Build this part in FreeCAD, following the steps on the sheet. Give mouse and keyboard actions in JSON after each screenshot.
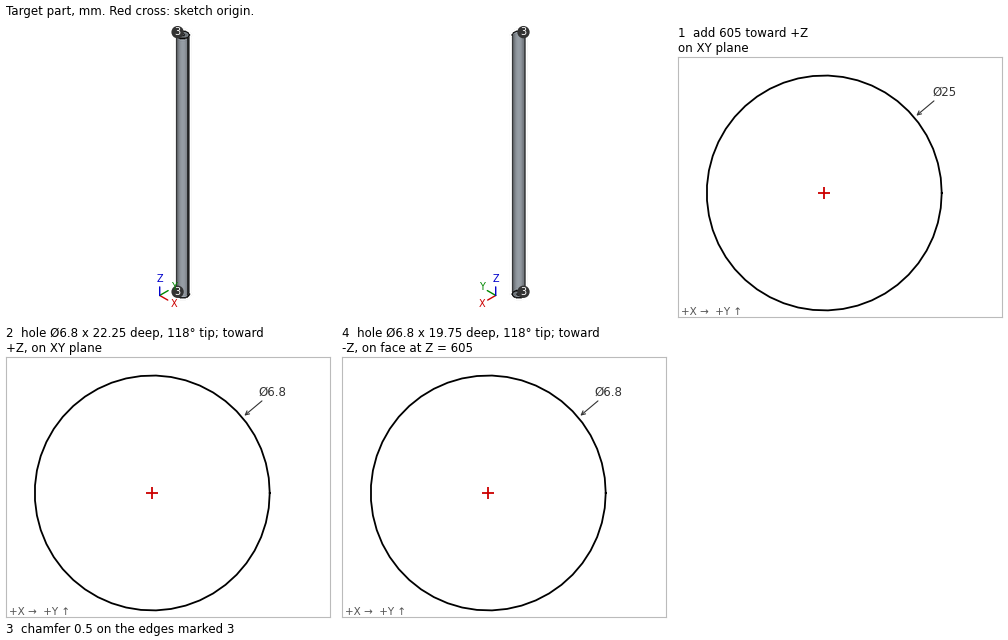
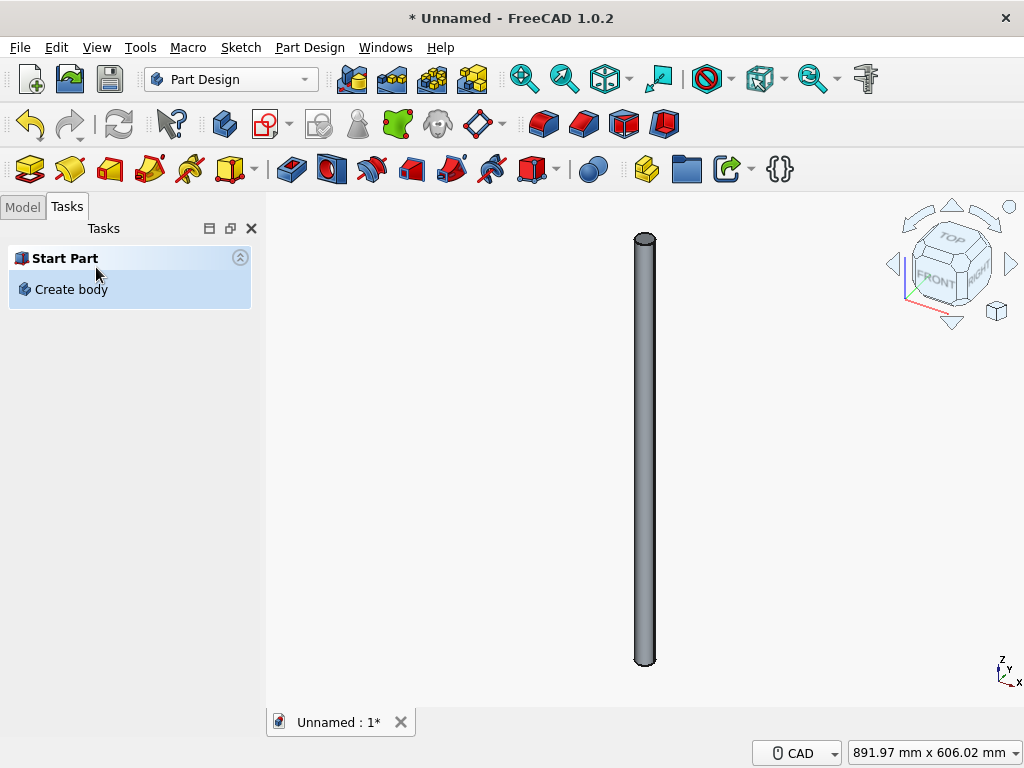
{"action": "key", "text": "0"}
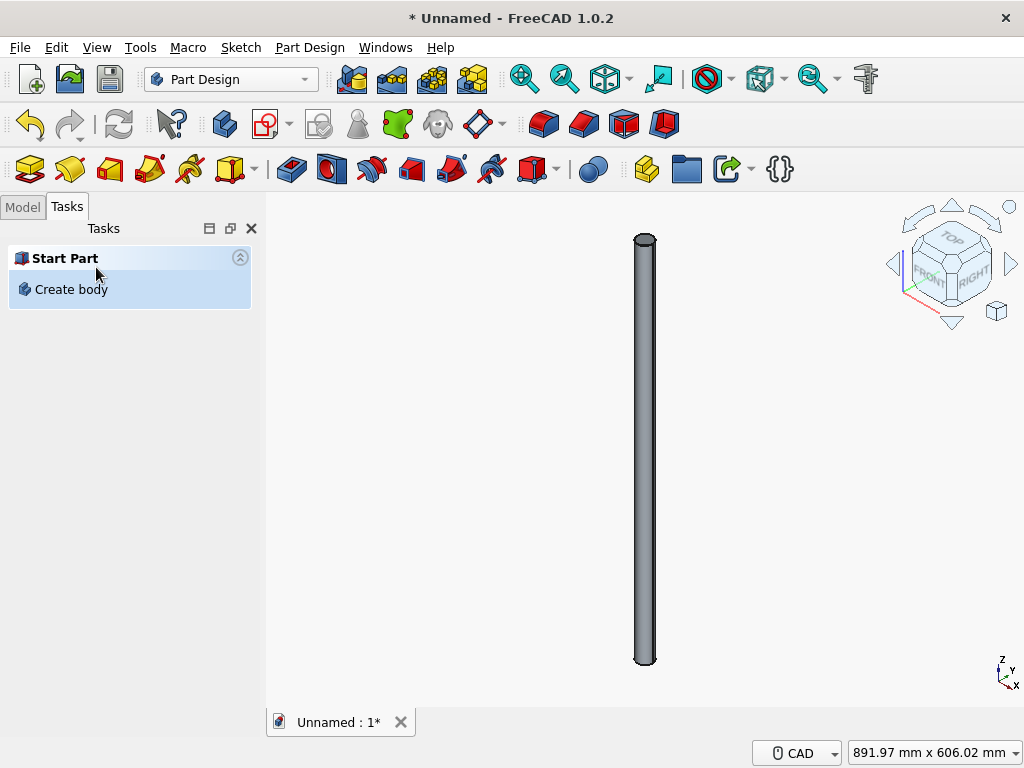
{"action": "key", "text": "2"}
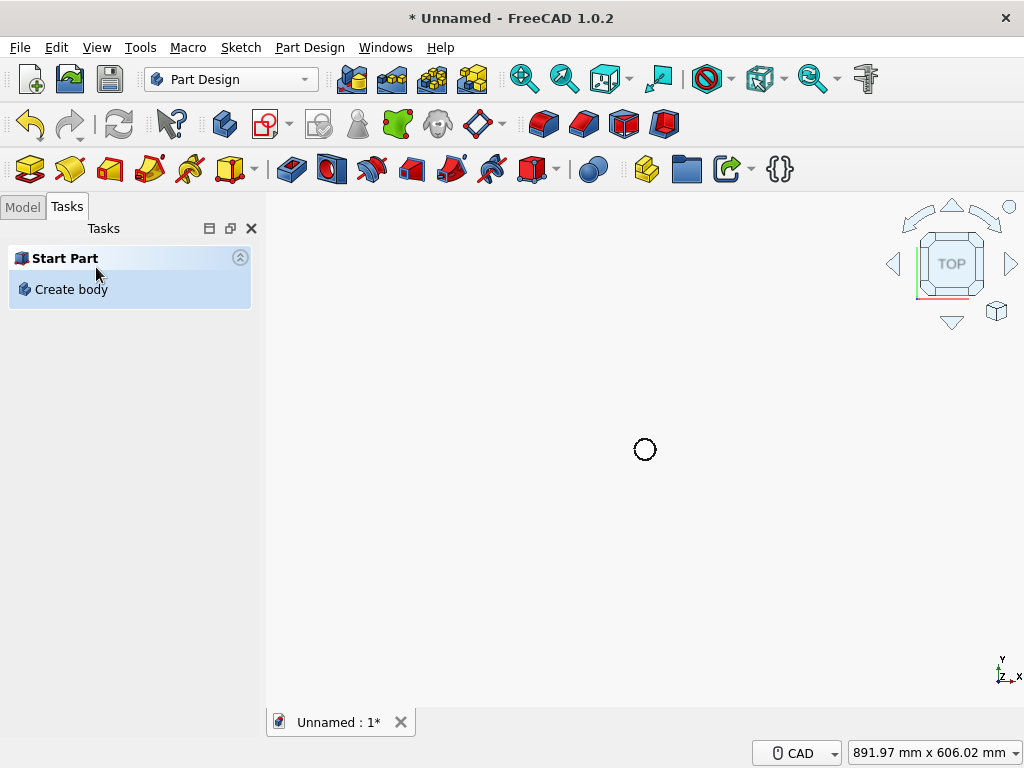
{"action": "left_click", "coordinate": [526, 80]}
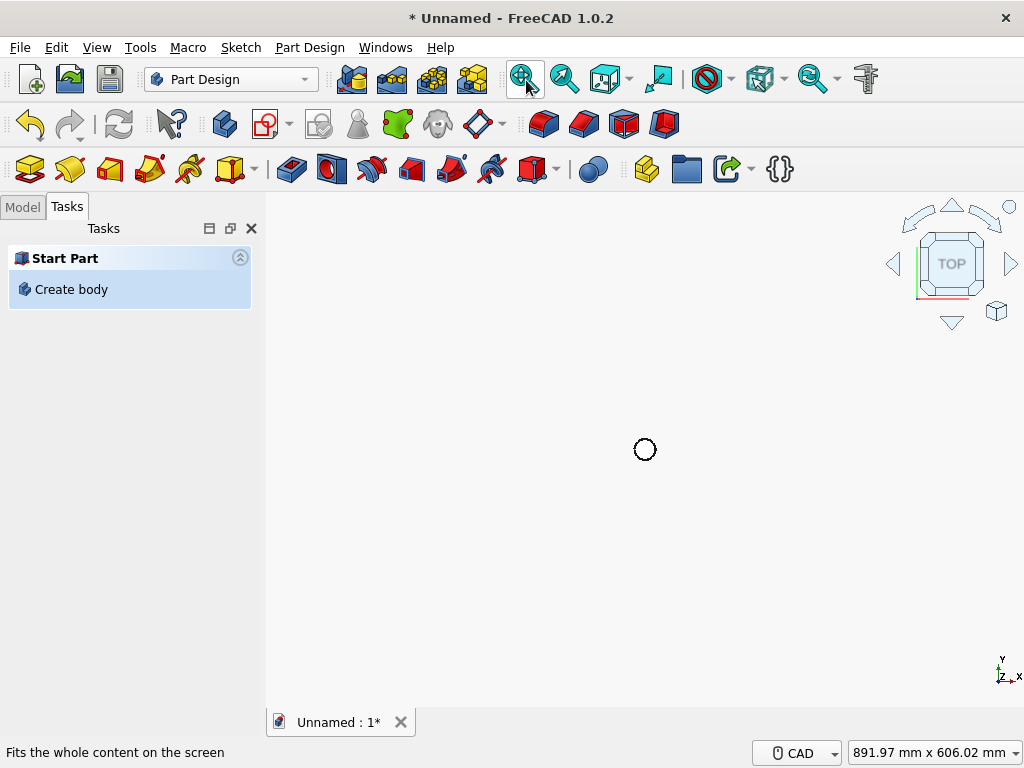
{"action": "left_click", "coordinate": [645, 448]}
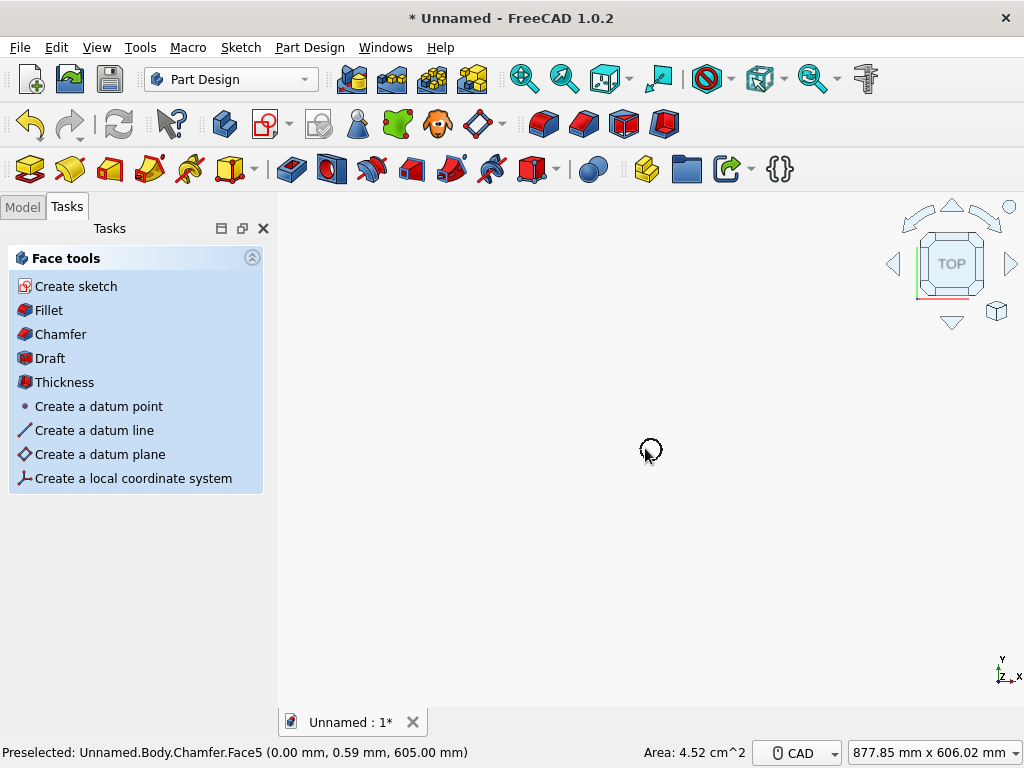
{"action": "left_click", "coordinate": [266, 124]}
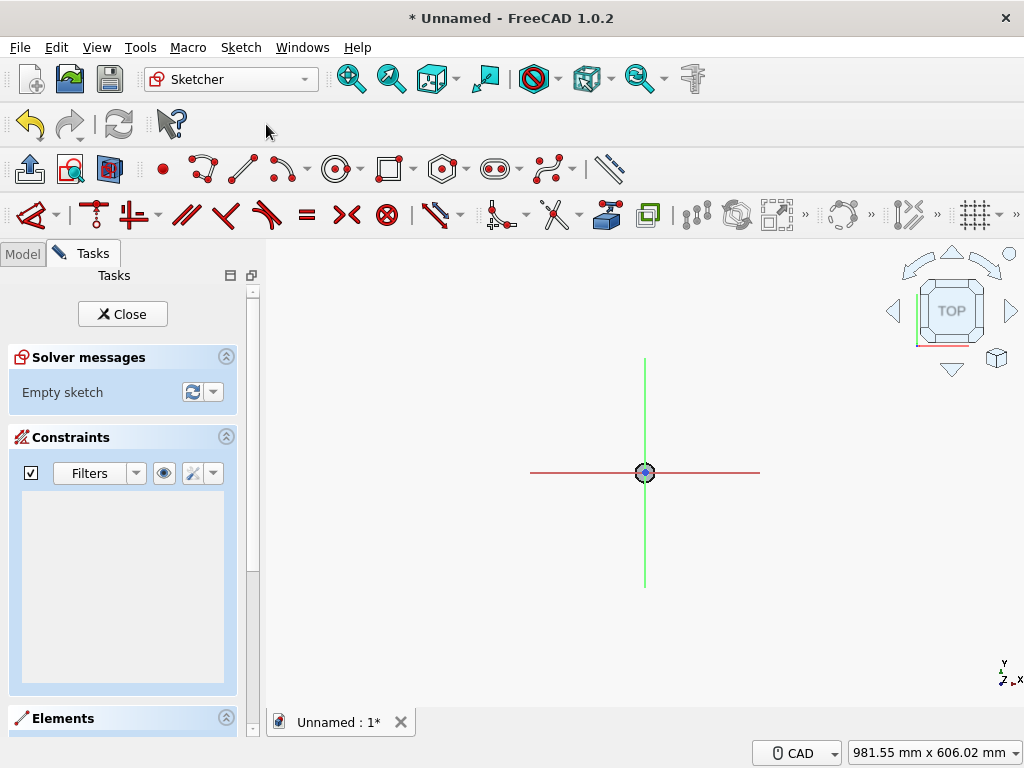
{"action": "scroll", "coordinate": [649, 473], "scroll_direction": "up", "scroll_amount": 15}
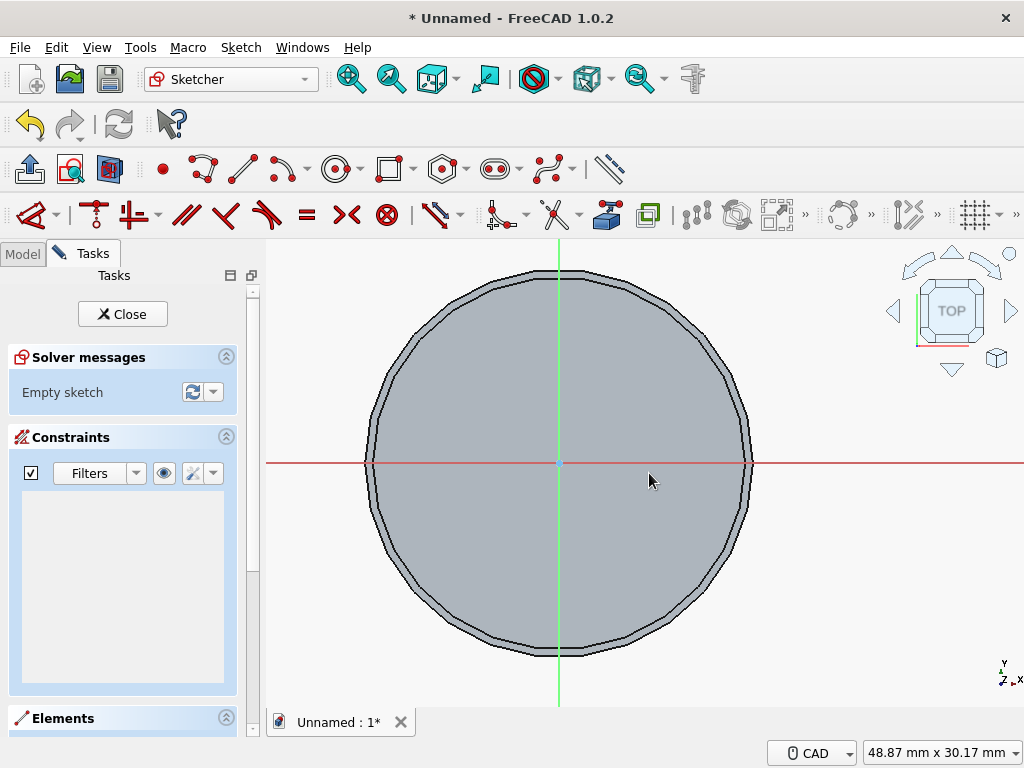
{"action": "scroll", "coordinate": [549, 458], "scroll_direction": "up", "scroll_amount": 5}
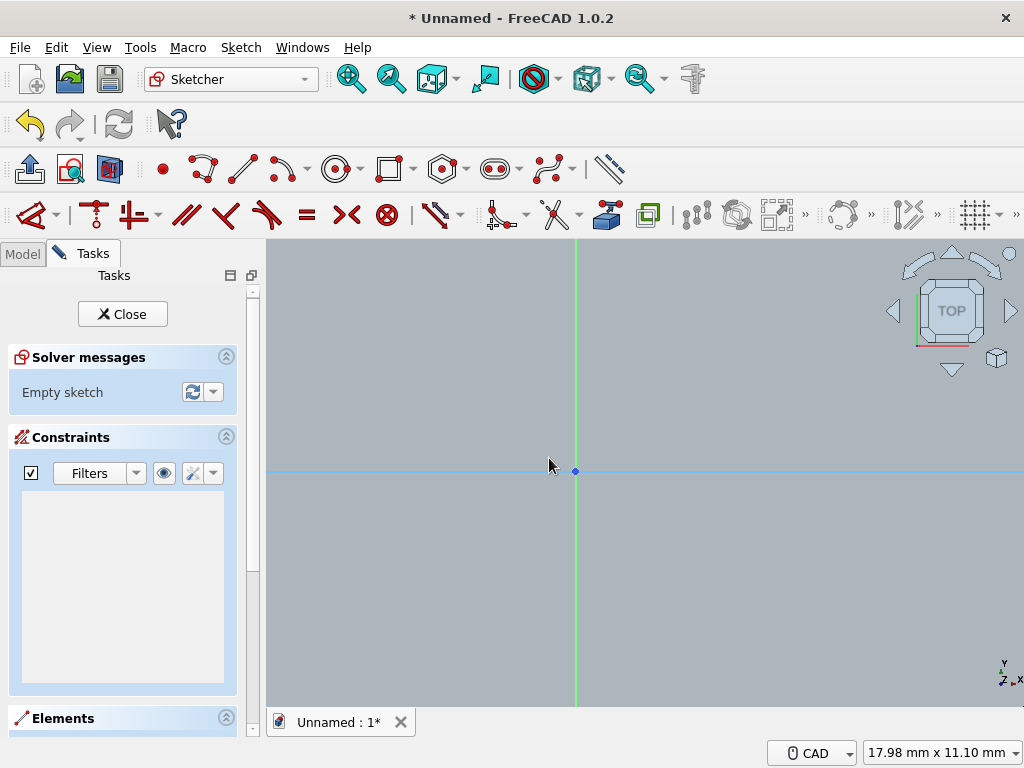
{"action": "left_click", "coordinate": [336, 170]}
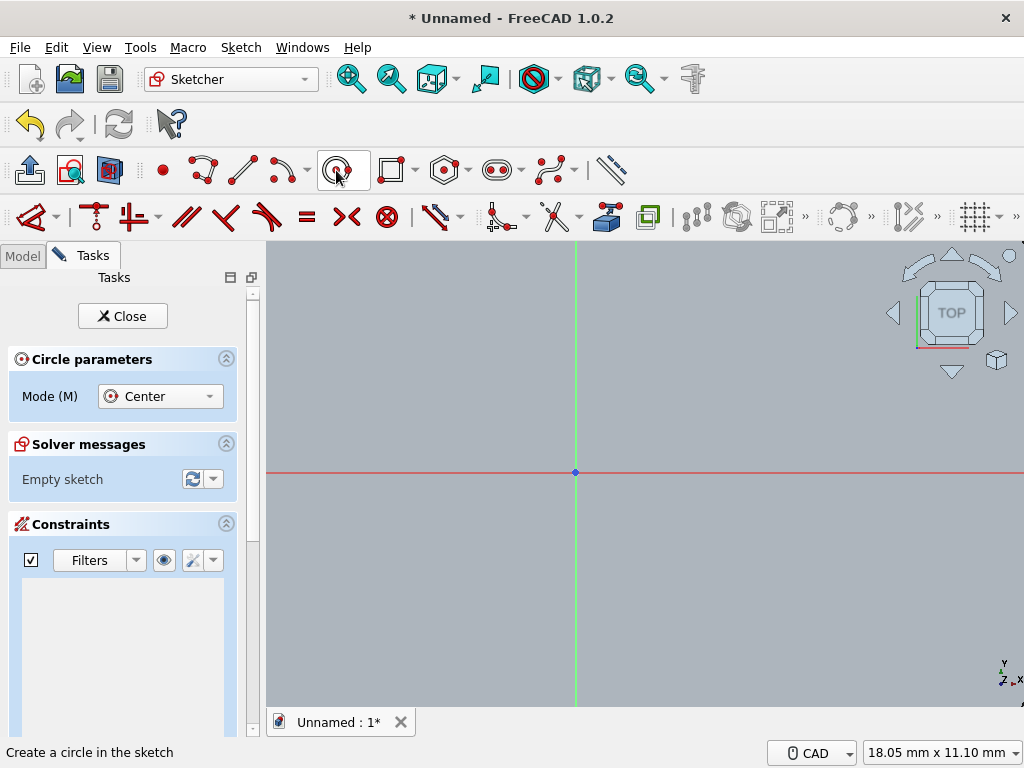
{"action": "left_click", "coordinate": [576, 473]}
{"action": "left_click", "coordinate": [677, 372]}
{"action": "key", "text": "Escape"}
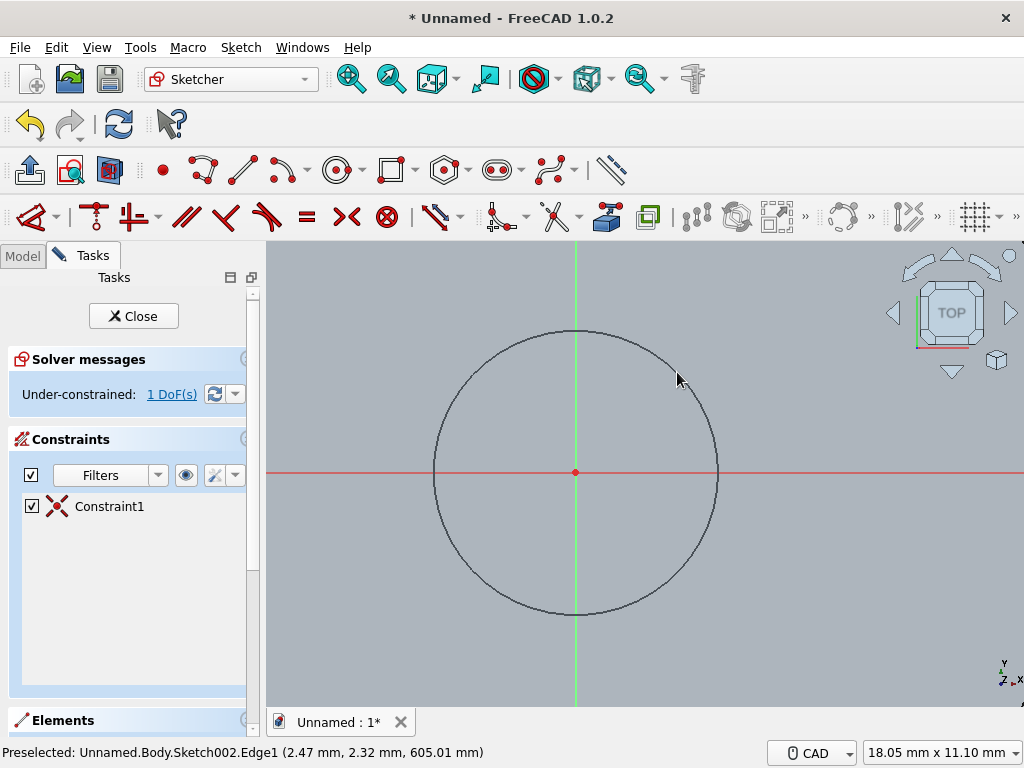
{"action": "left_click", "coordinate": [32, 218]}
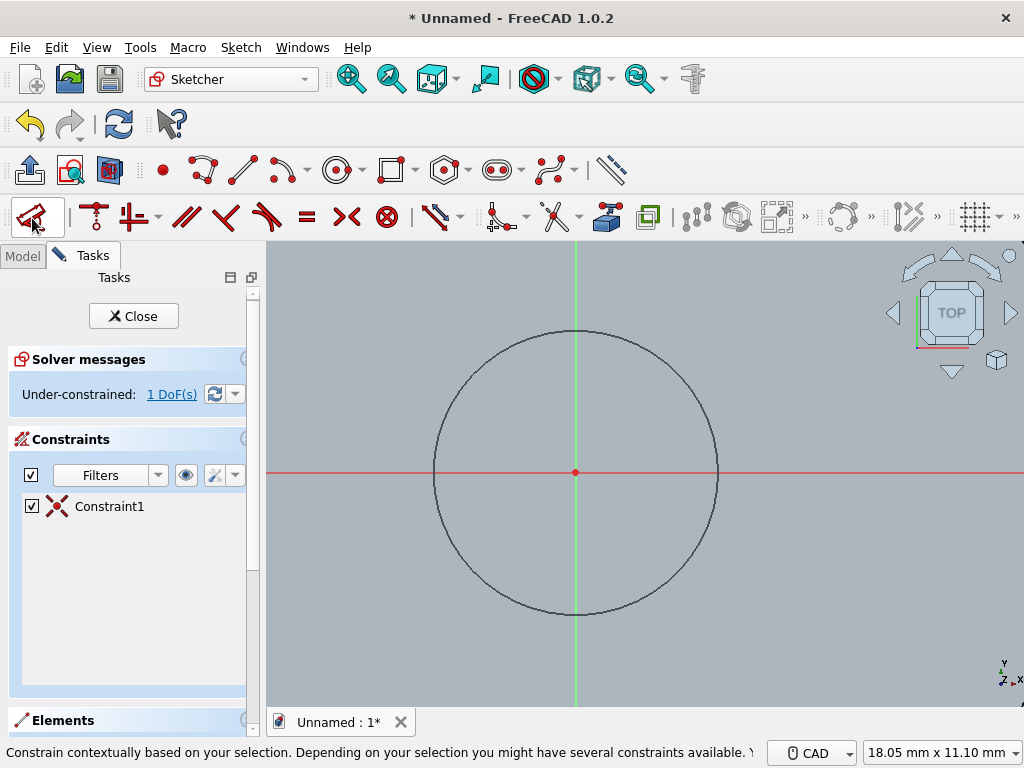
{"action": "left_click", "coordinate": [676, 372]}
{"action": "left_click", "coordinate": [699, 349]}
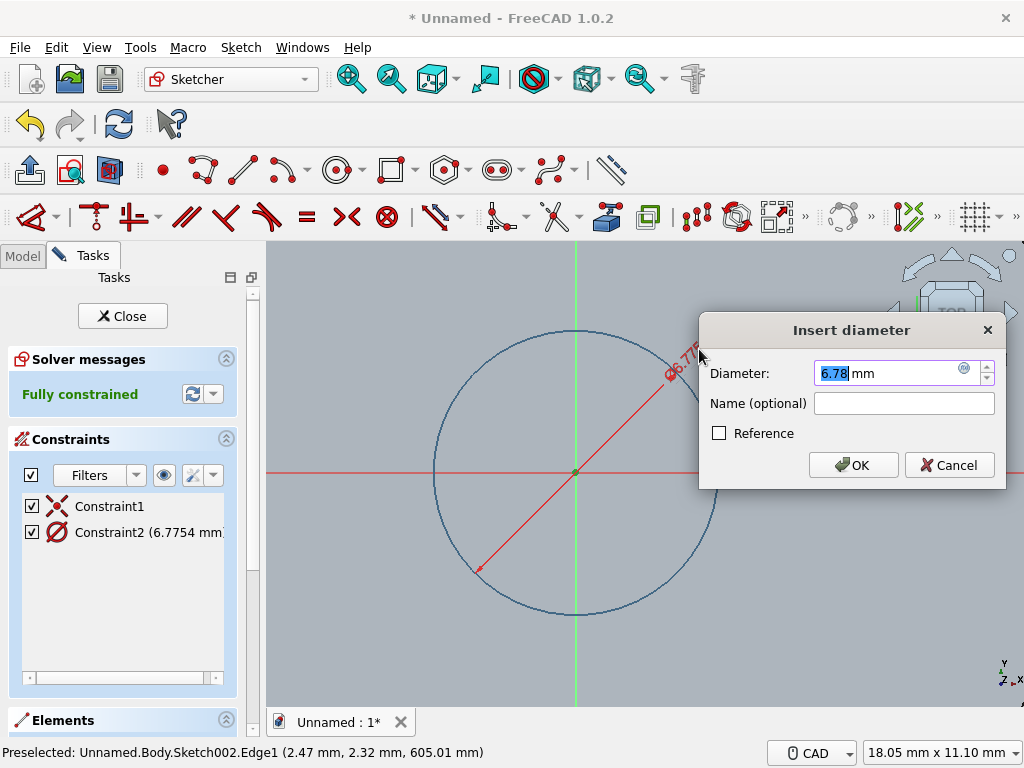
{"action": "type", "text": "6.8"}
{"action": "key", "text": "Return"}
{"action": "key", "text": "Escape"}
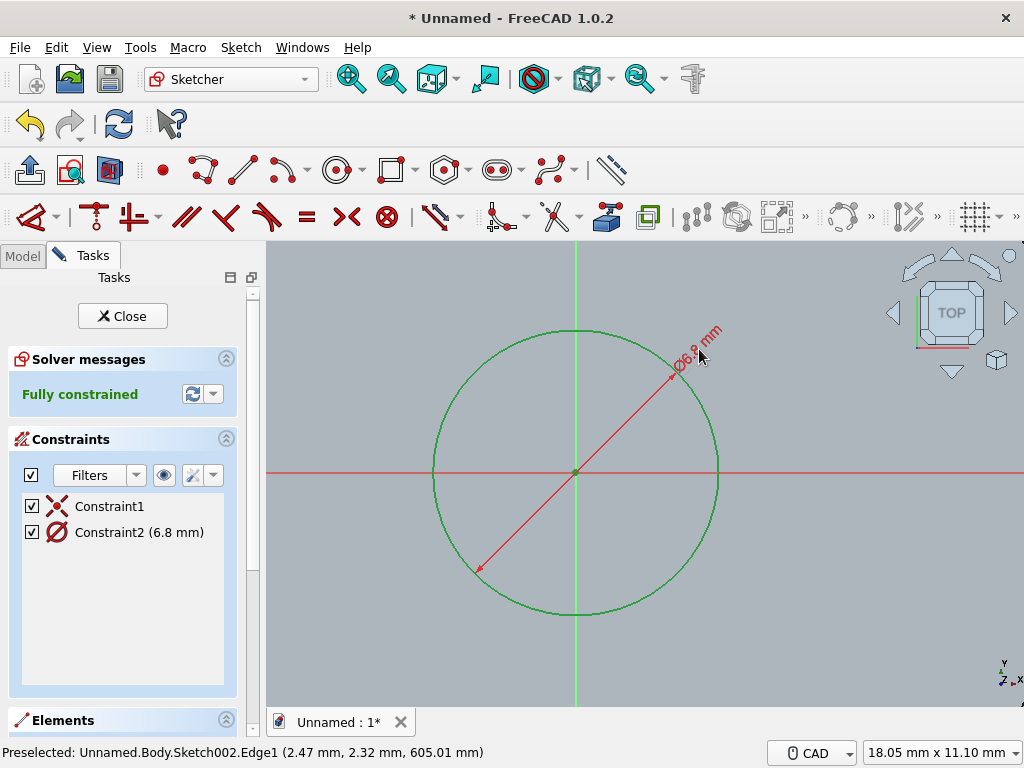
{"action": "left_click", "coordinate": [123, 316]}